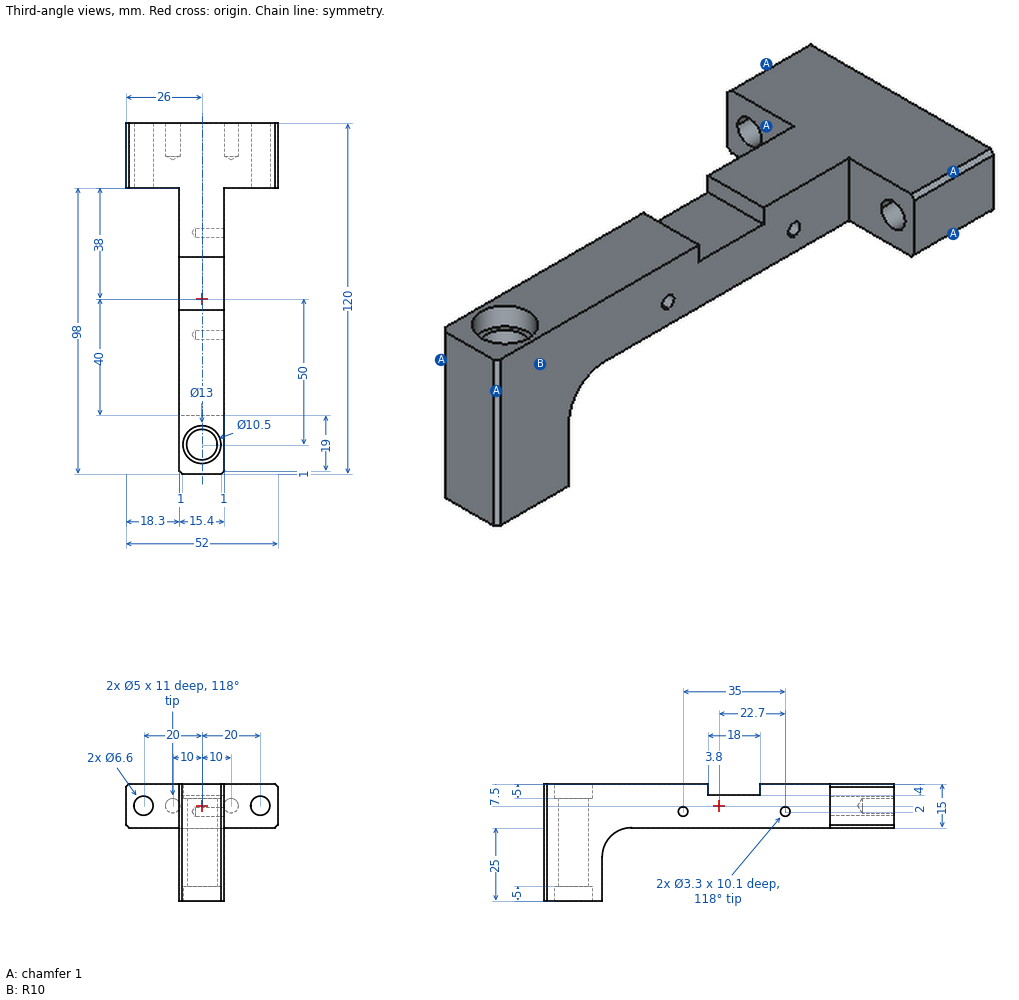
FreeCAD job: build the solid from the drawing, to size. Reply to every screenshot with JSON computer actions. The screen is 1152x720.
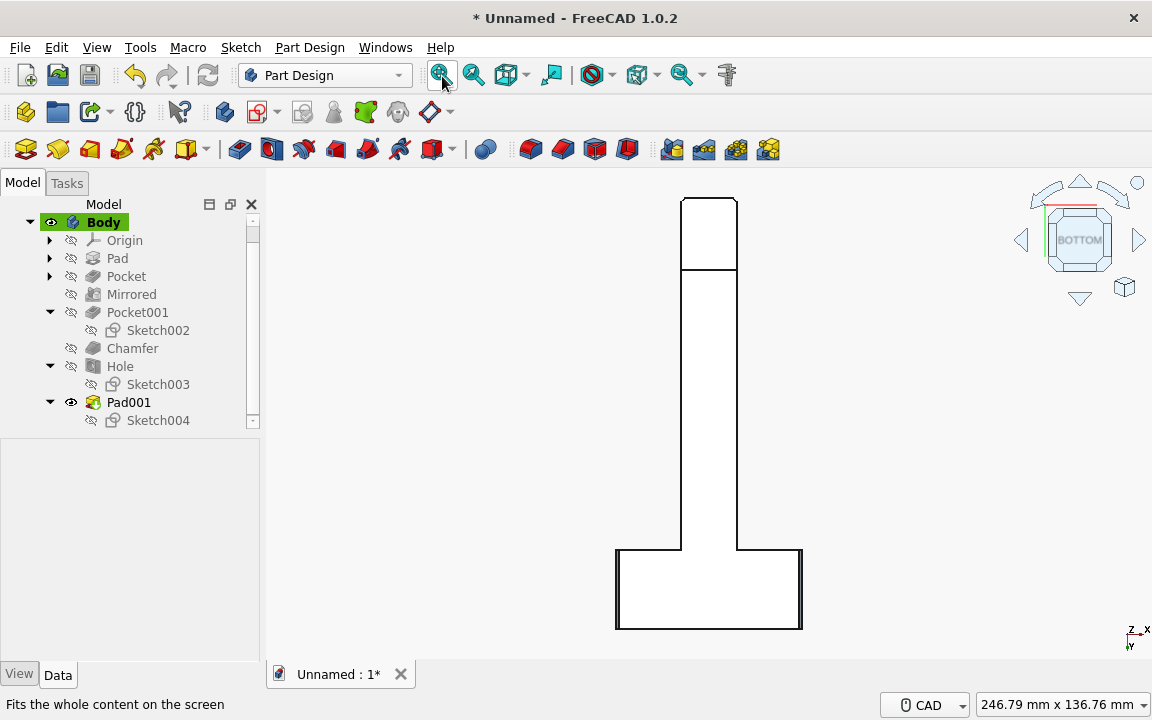
{"action": "key", "text": "4"}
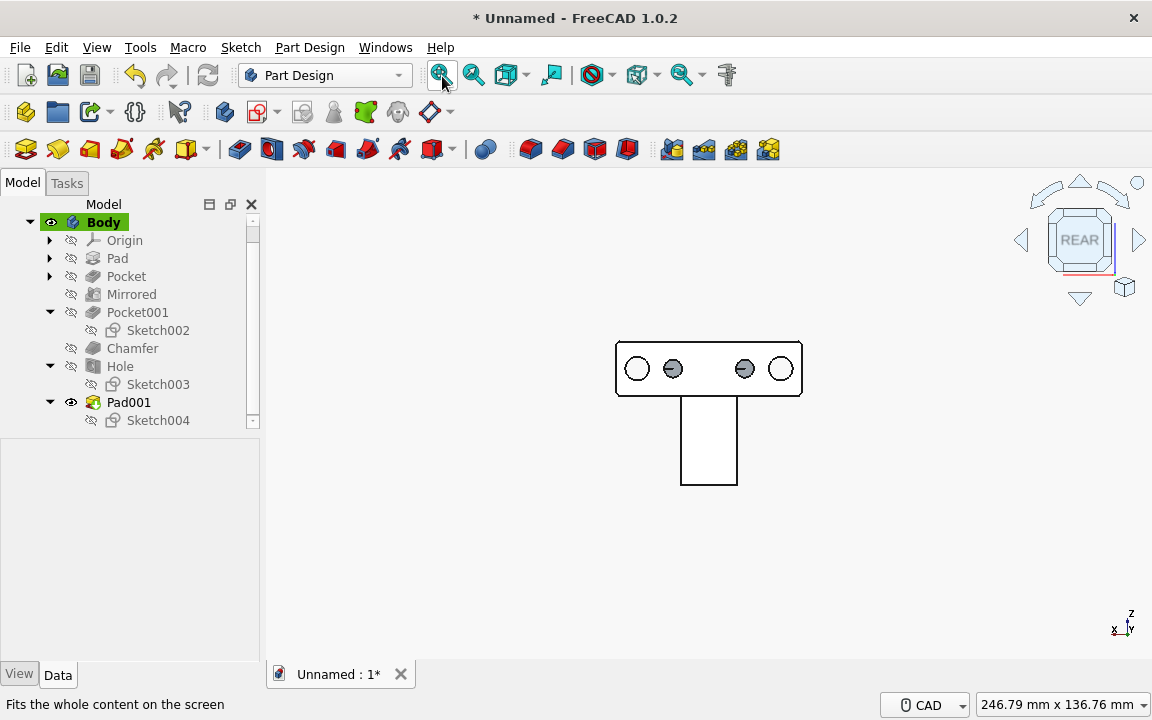
{"action": "left_click", "coordinate": [442, 76]}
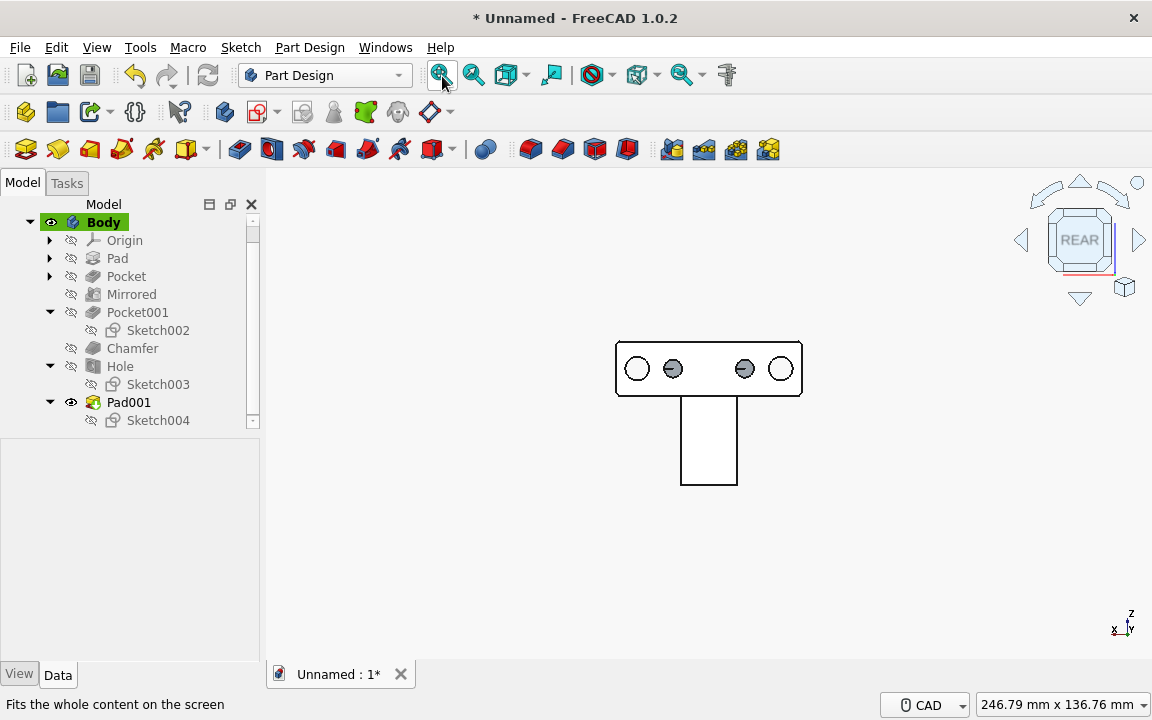
{"action": "key", "text": "6"}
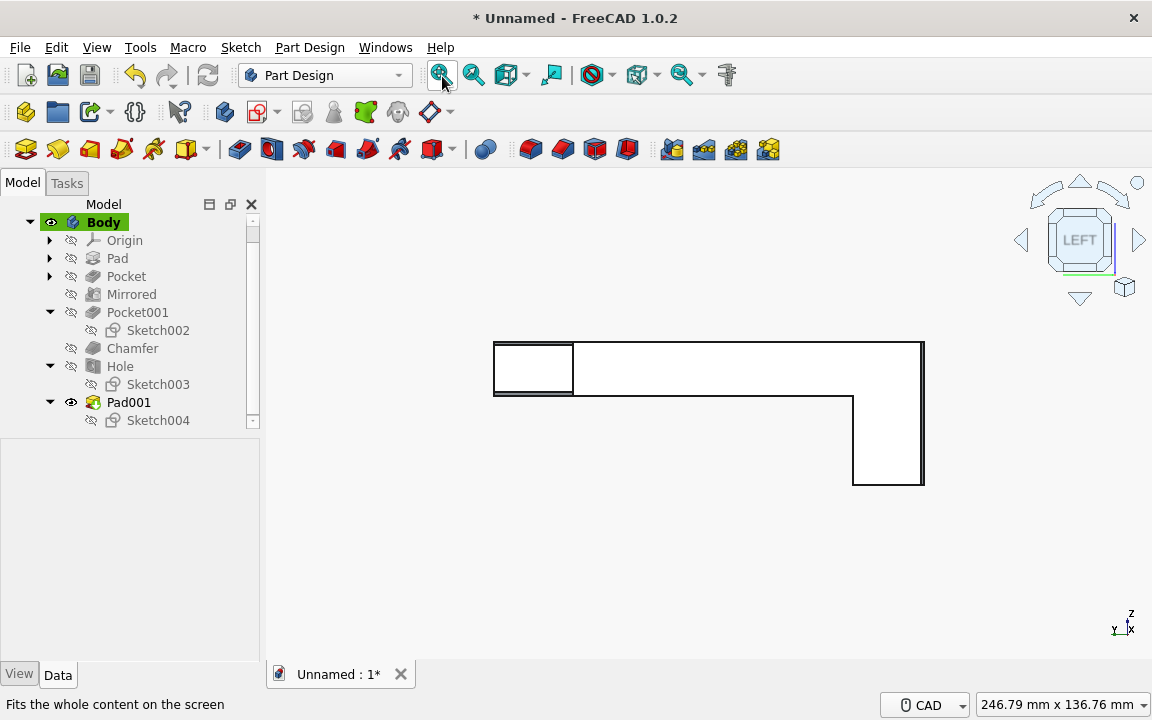
{"action": "key", "text": "v 3"}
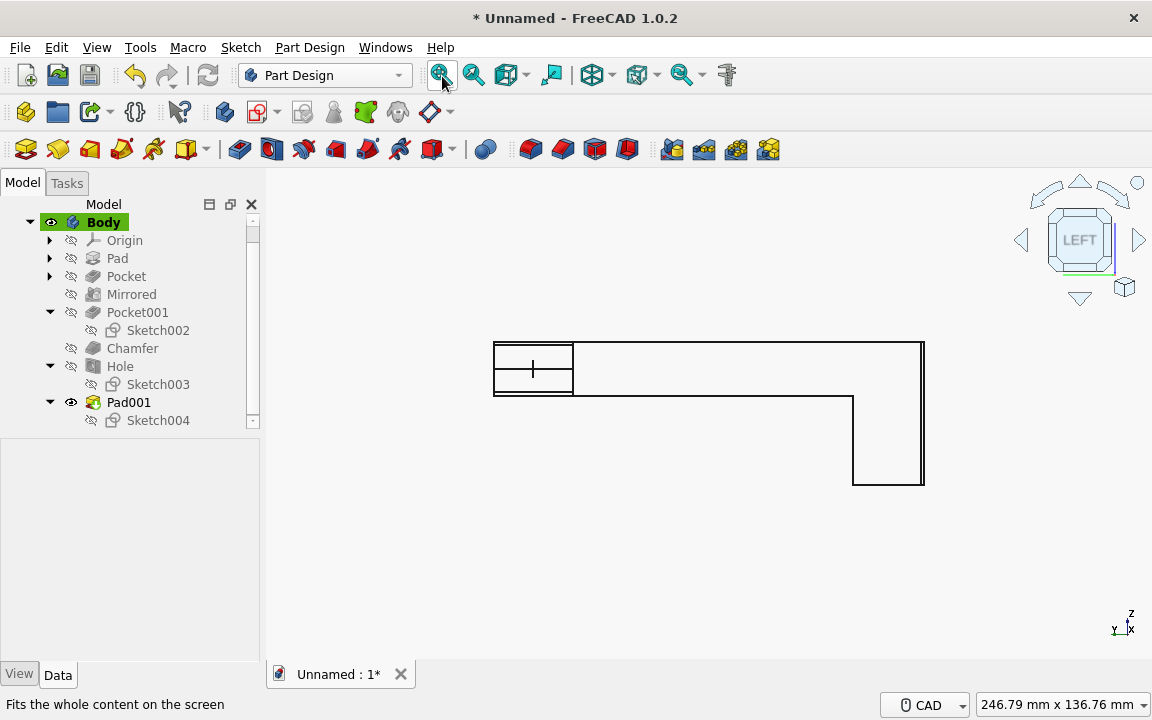
{"action": "key", "text": "0"}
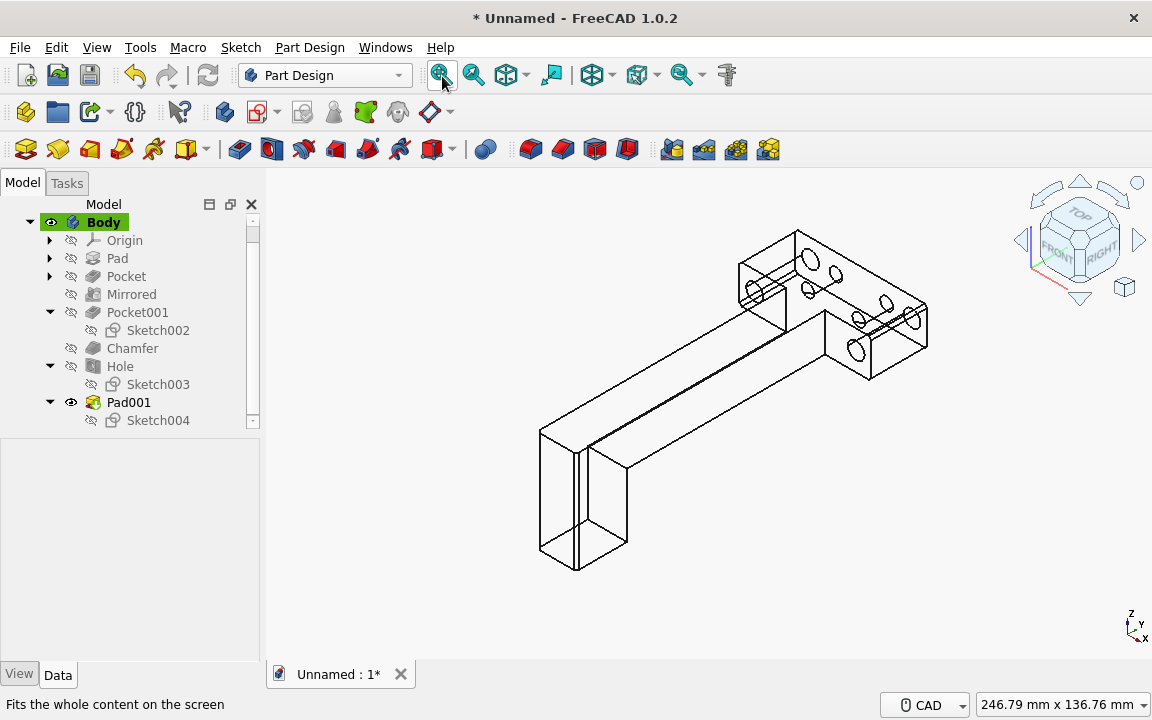
{"action": "left_click", "coordinate": [607, 456]}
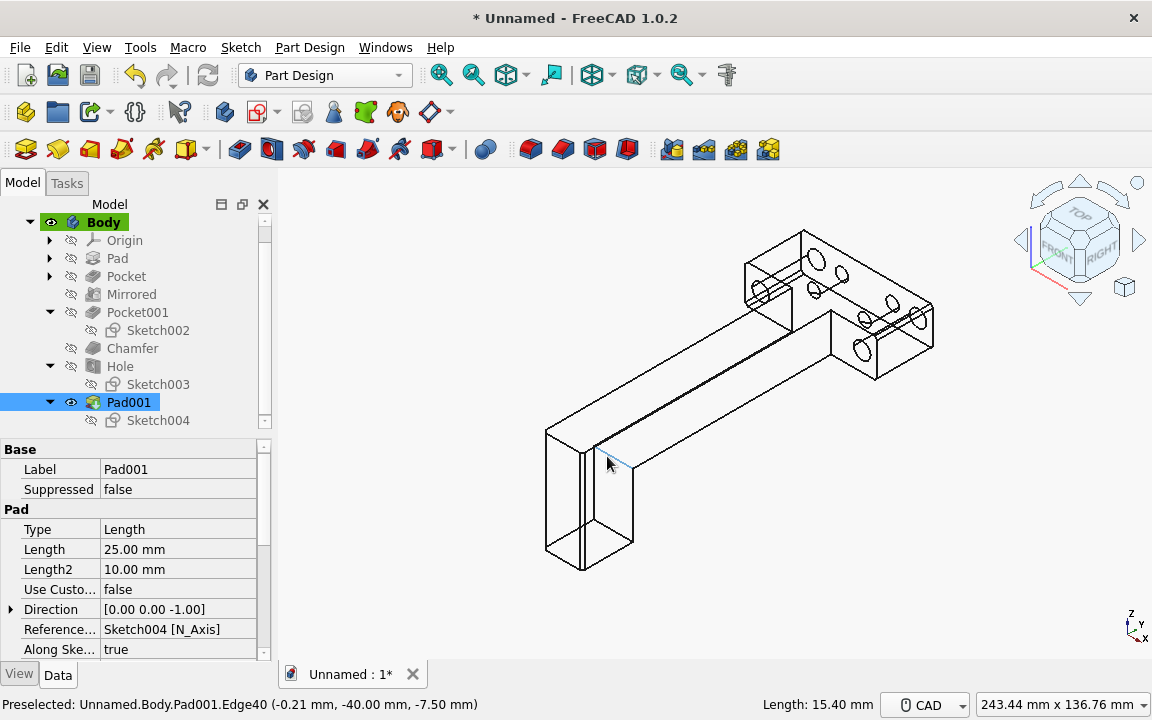
{"action": "key", "text": "v 1"}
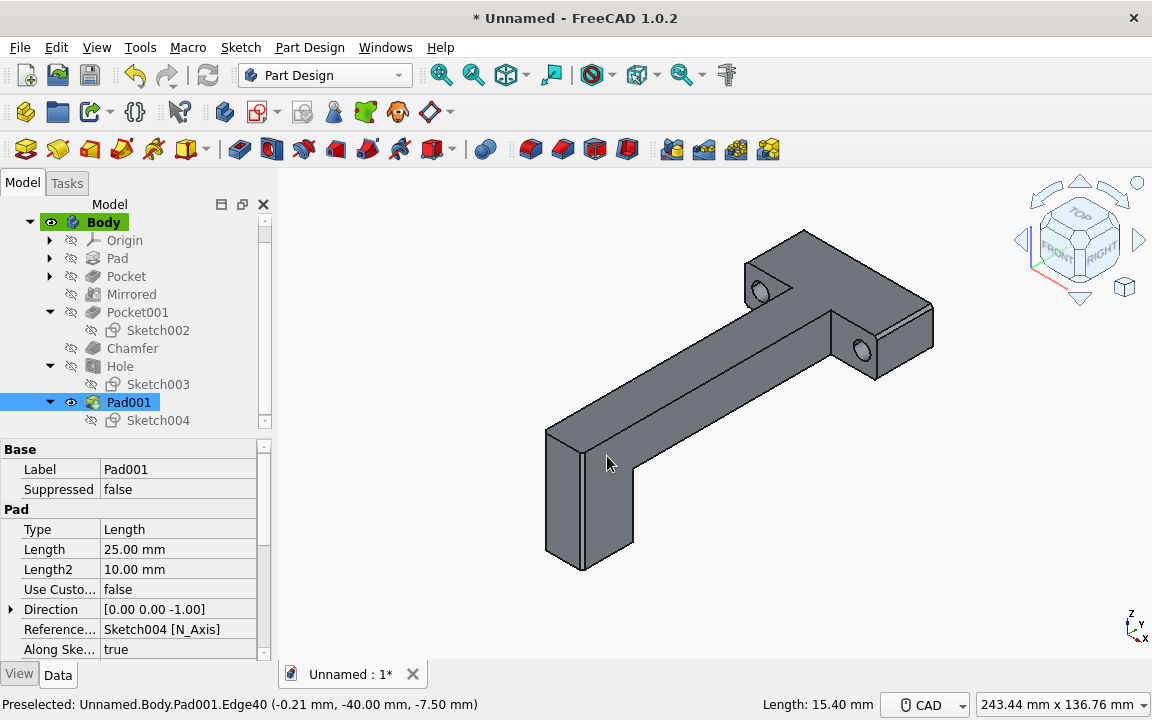
{"action": "left_click", "coordinate": [532, 150]}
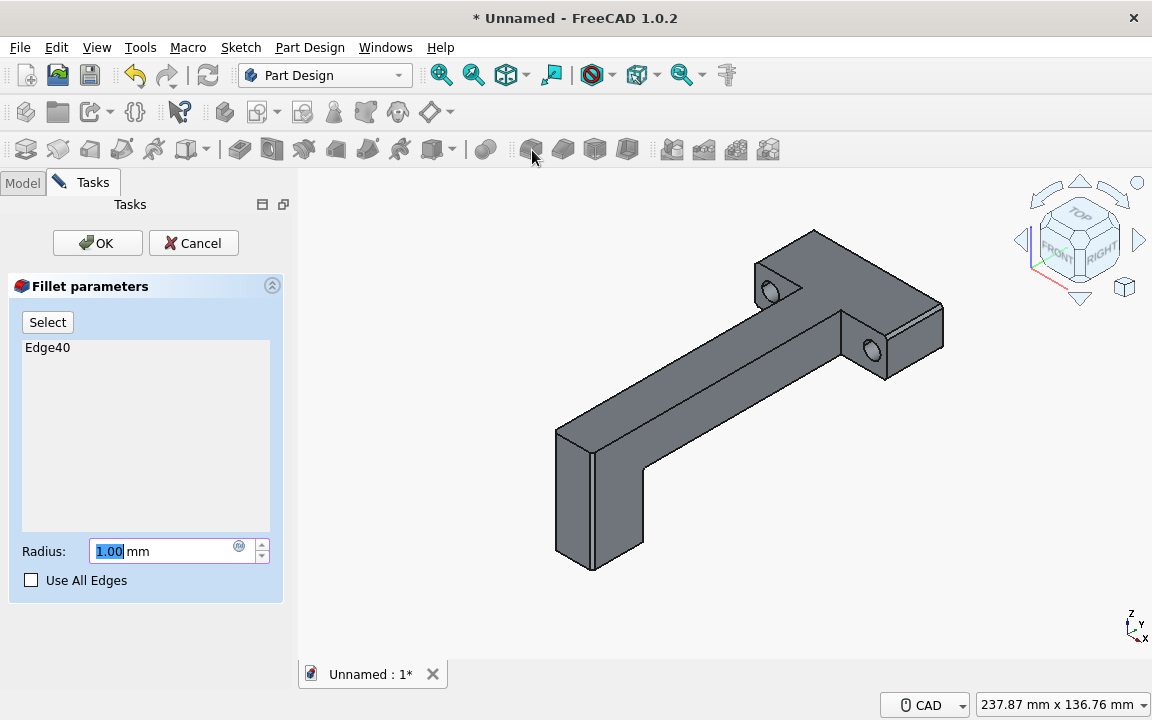
{"action": "type", "text": "10"}
{"action": "key", "text": "Tab"}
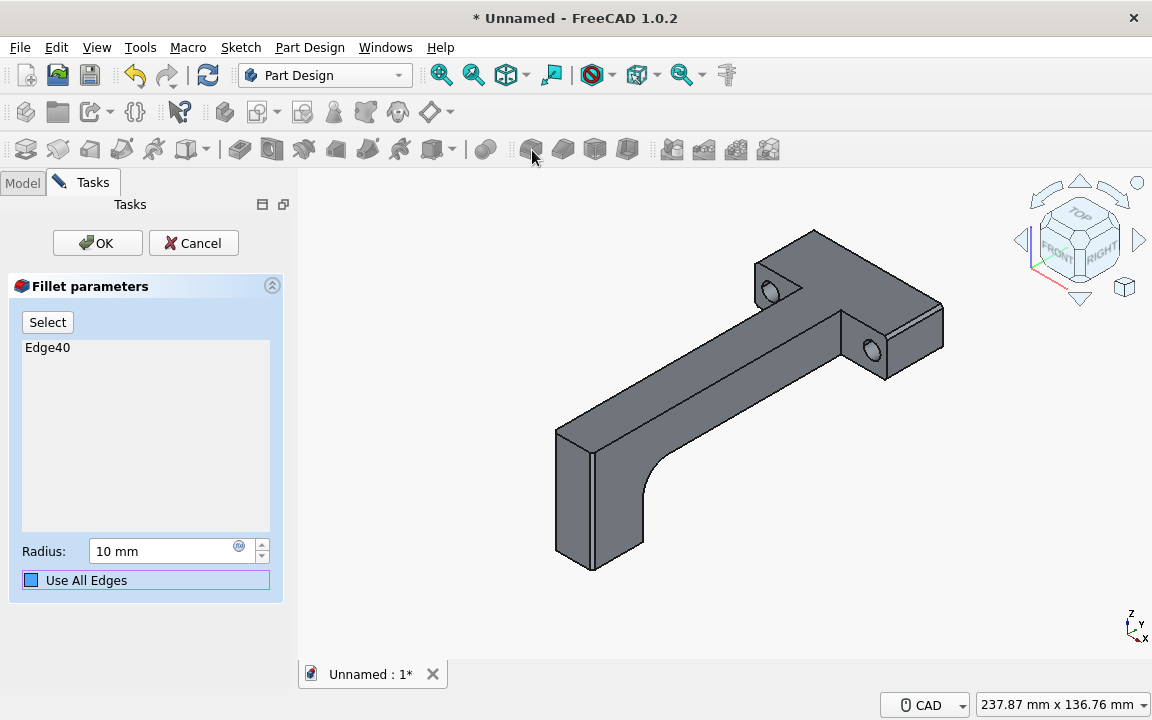
{"action": "left_click", "coordinate": [98, 243]}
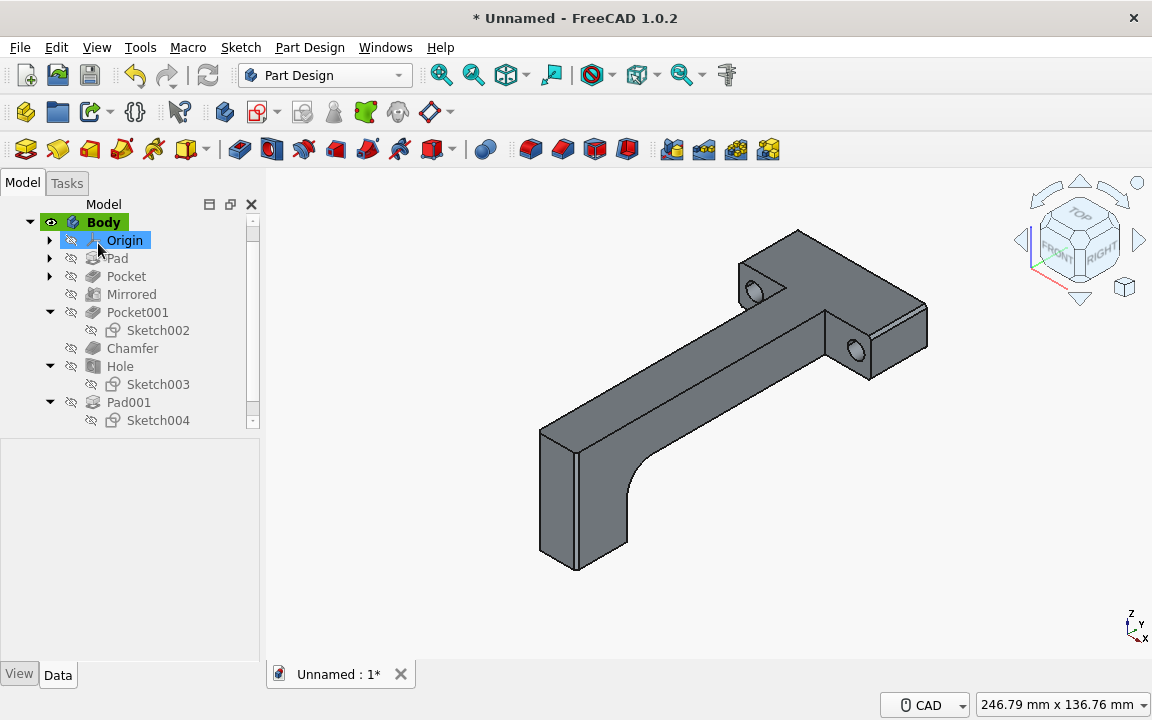
{"action": "left_click", "coordinate": [876, 299]}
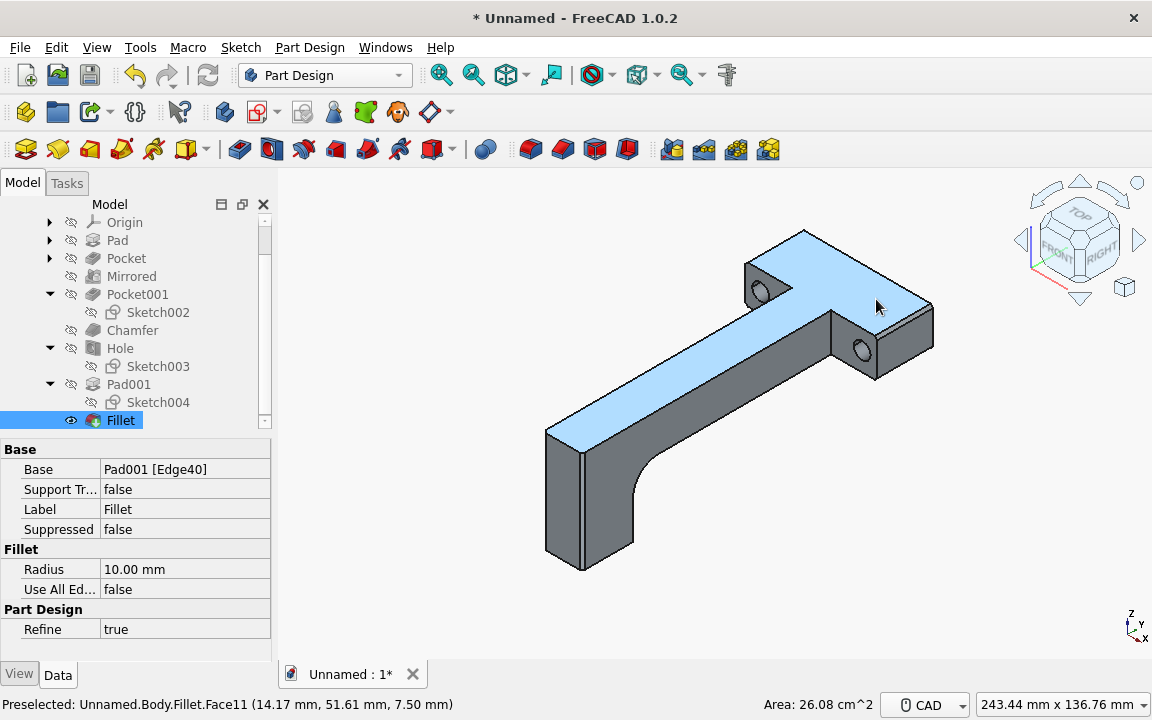
{"action": "left_click", "coordinate": [258, 112]}